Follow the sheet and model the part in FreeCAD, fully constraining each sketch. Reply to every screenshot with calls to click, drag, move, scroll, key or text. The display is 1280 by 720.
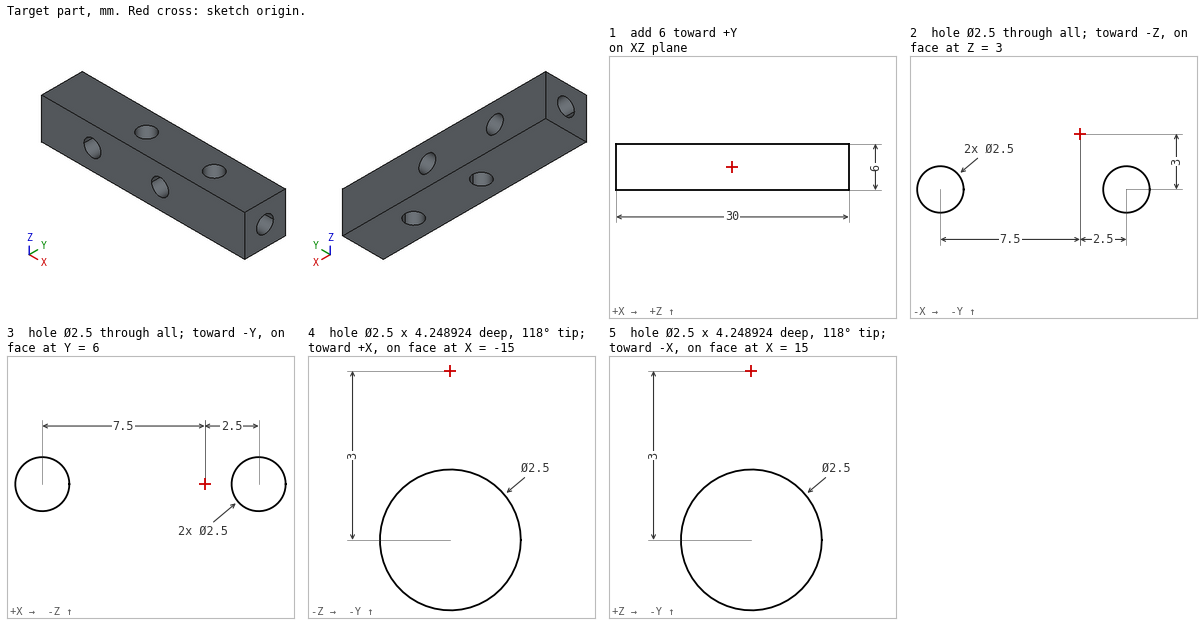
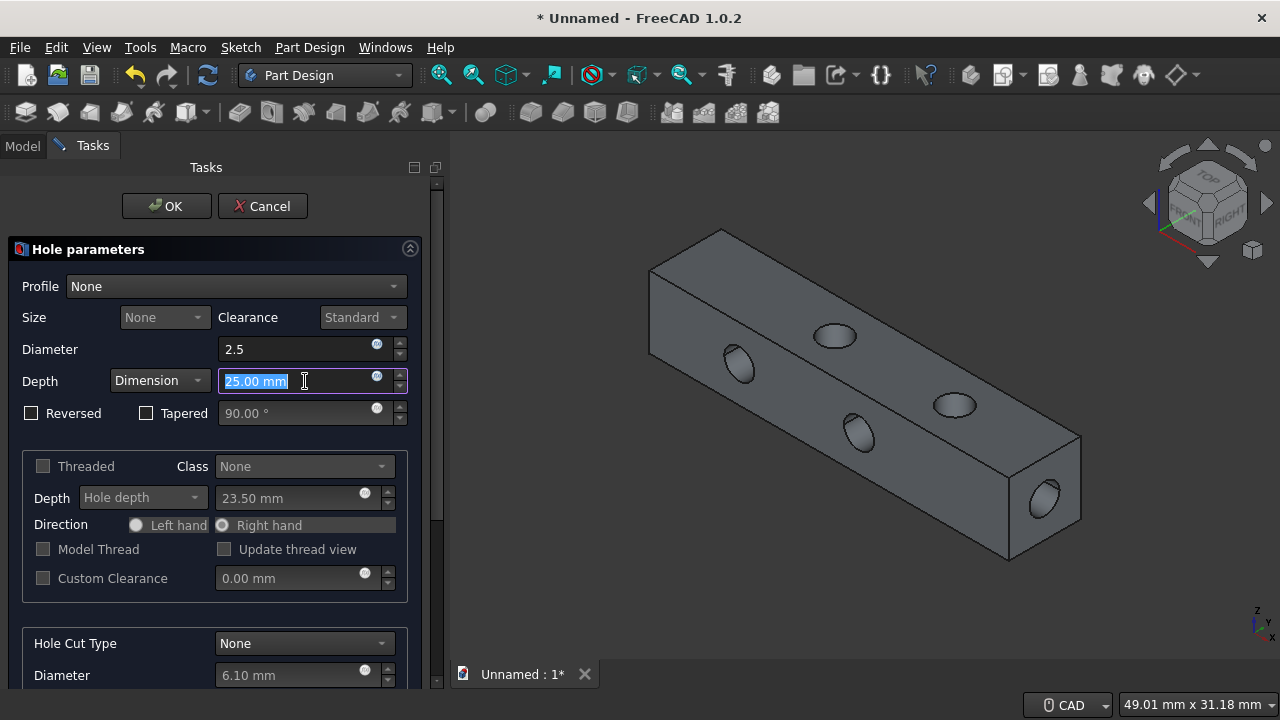
text(4.248924)
key(Tab)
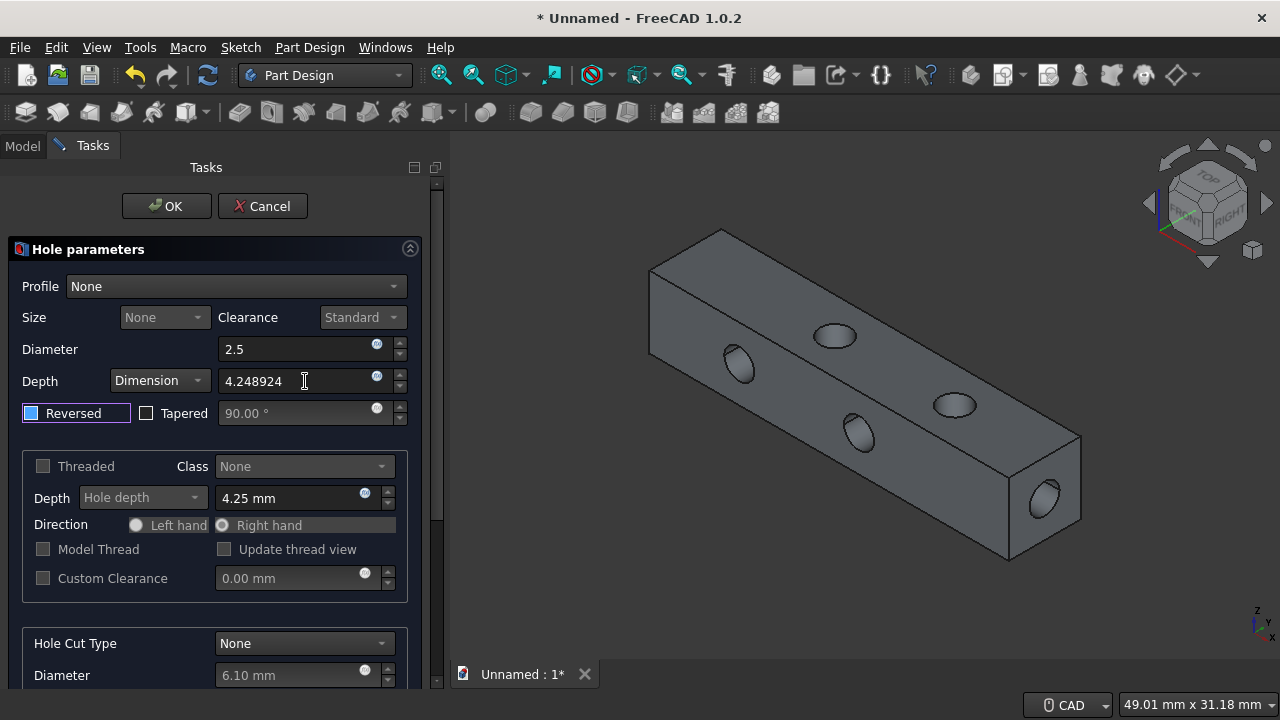
click(167, 206)